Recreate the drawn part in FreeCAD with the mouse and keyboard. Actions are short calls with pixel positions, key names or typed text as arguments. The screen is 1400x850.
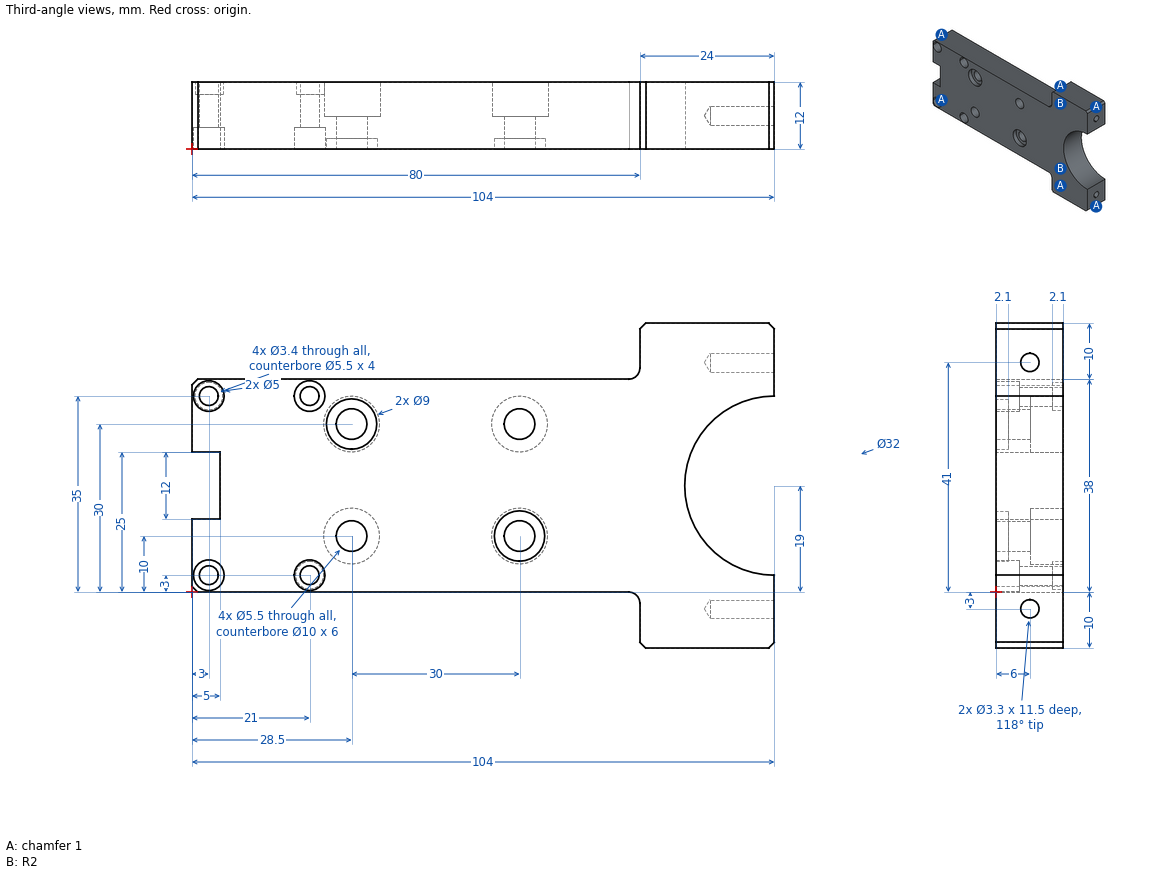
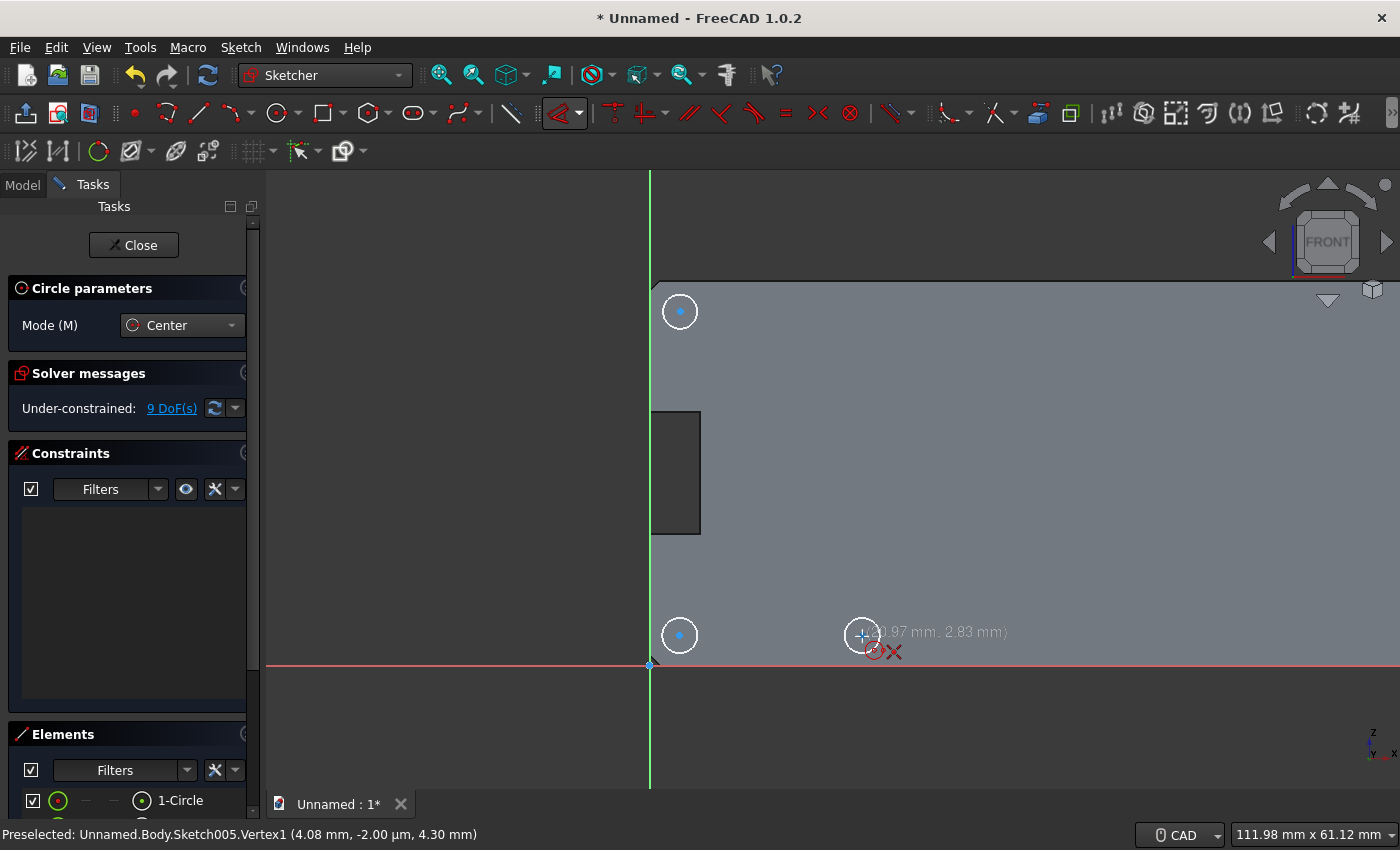
scroll(862, 311, up, 2)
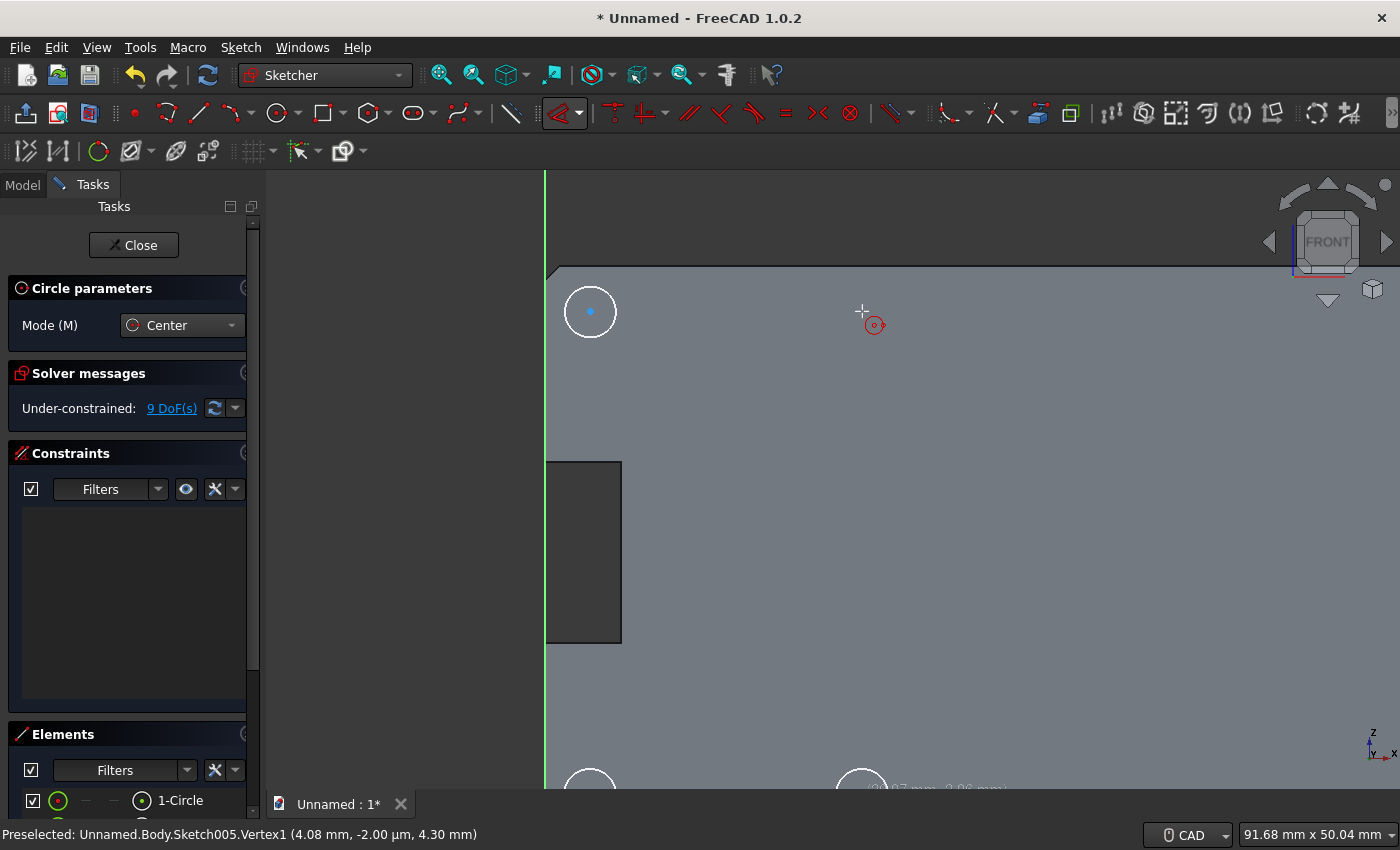
click(862, 311)
click(881, 293)
key(Escape)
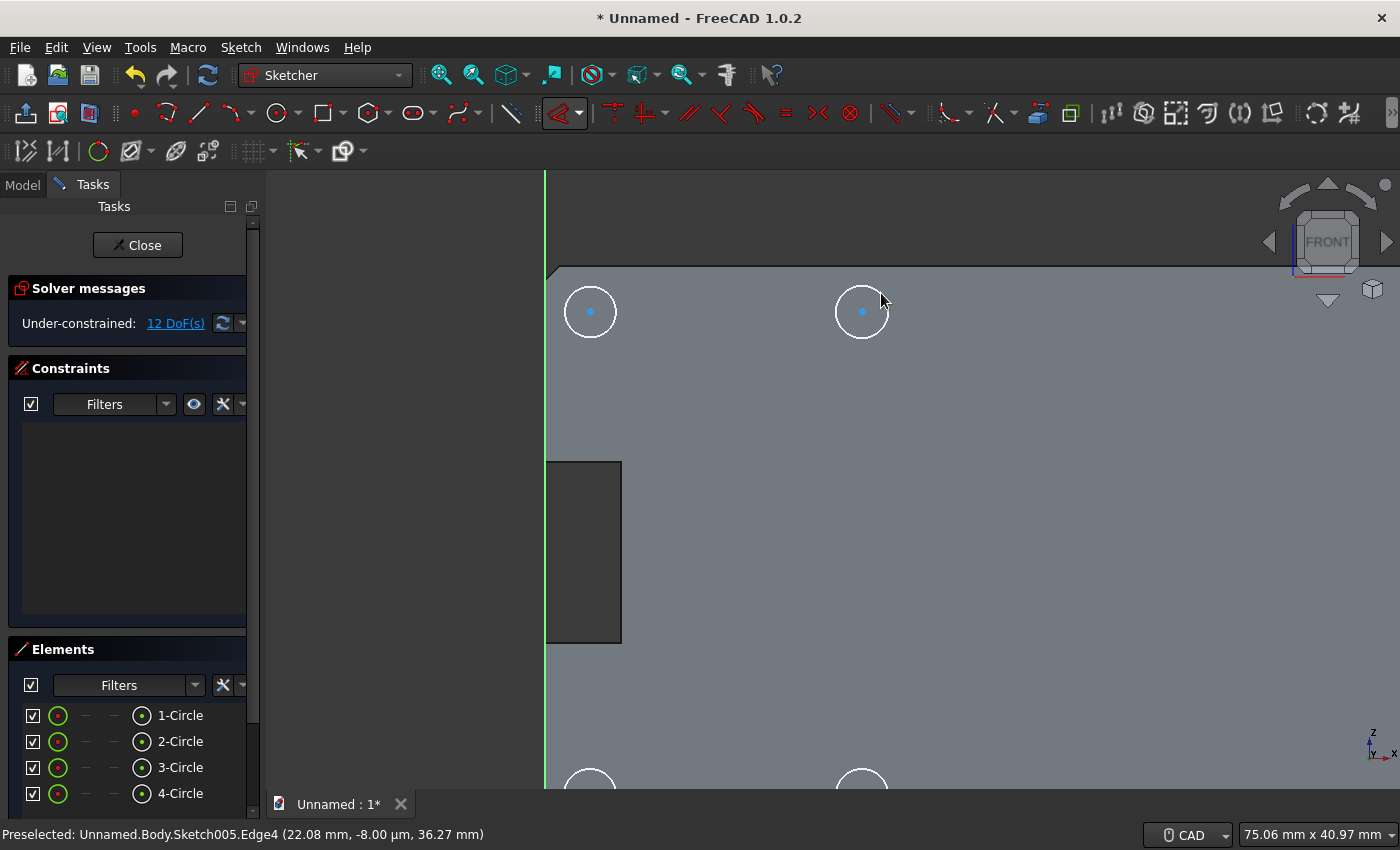
click(608, 294)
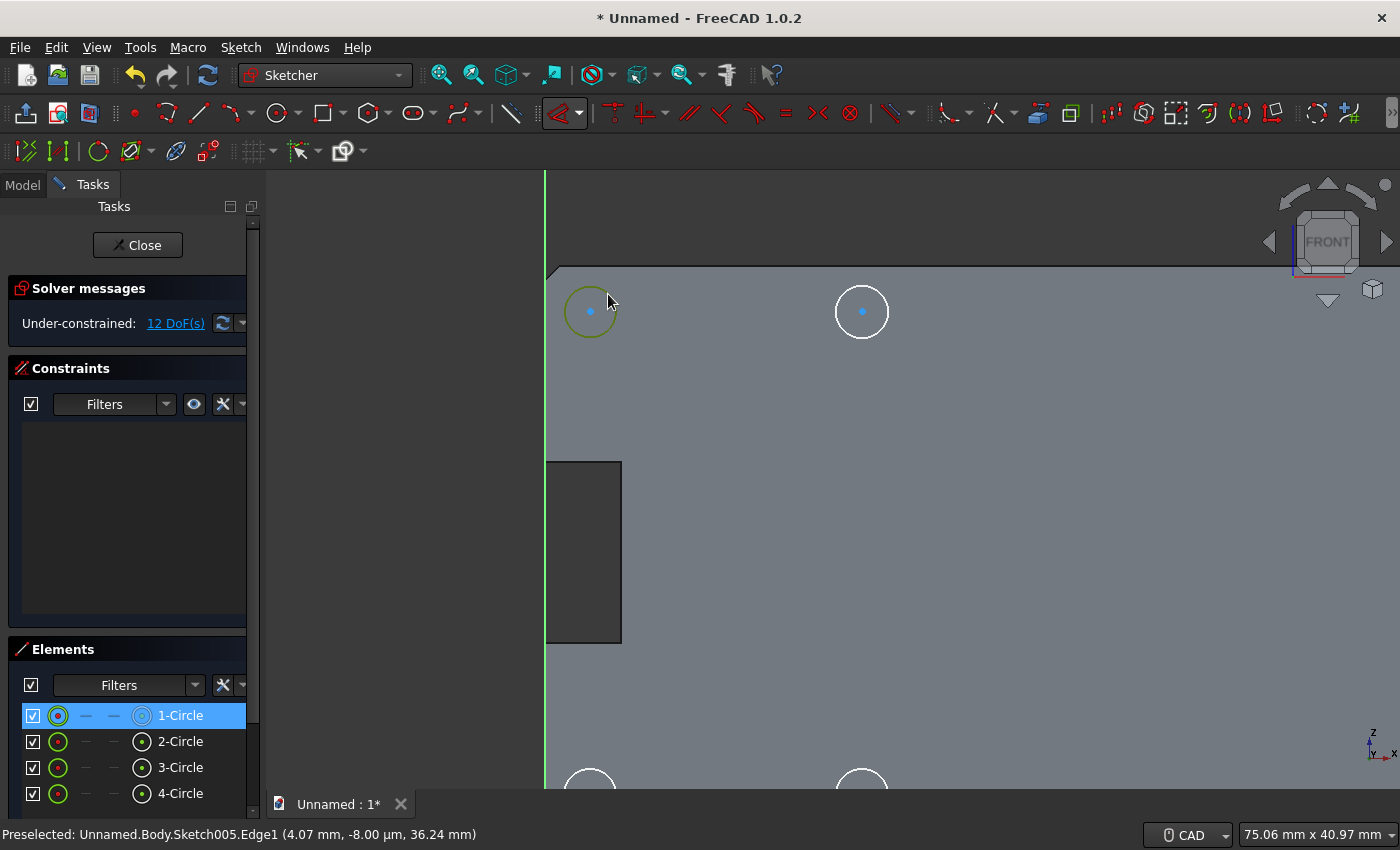
scroll(862, 310, down, 2)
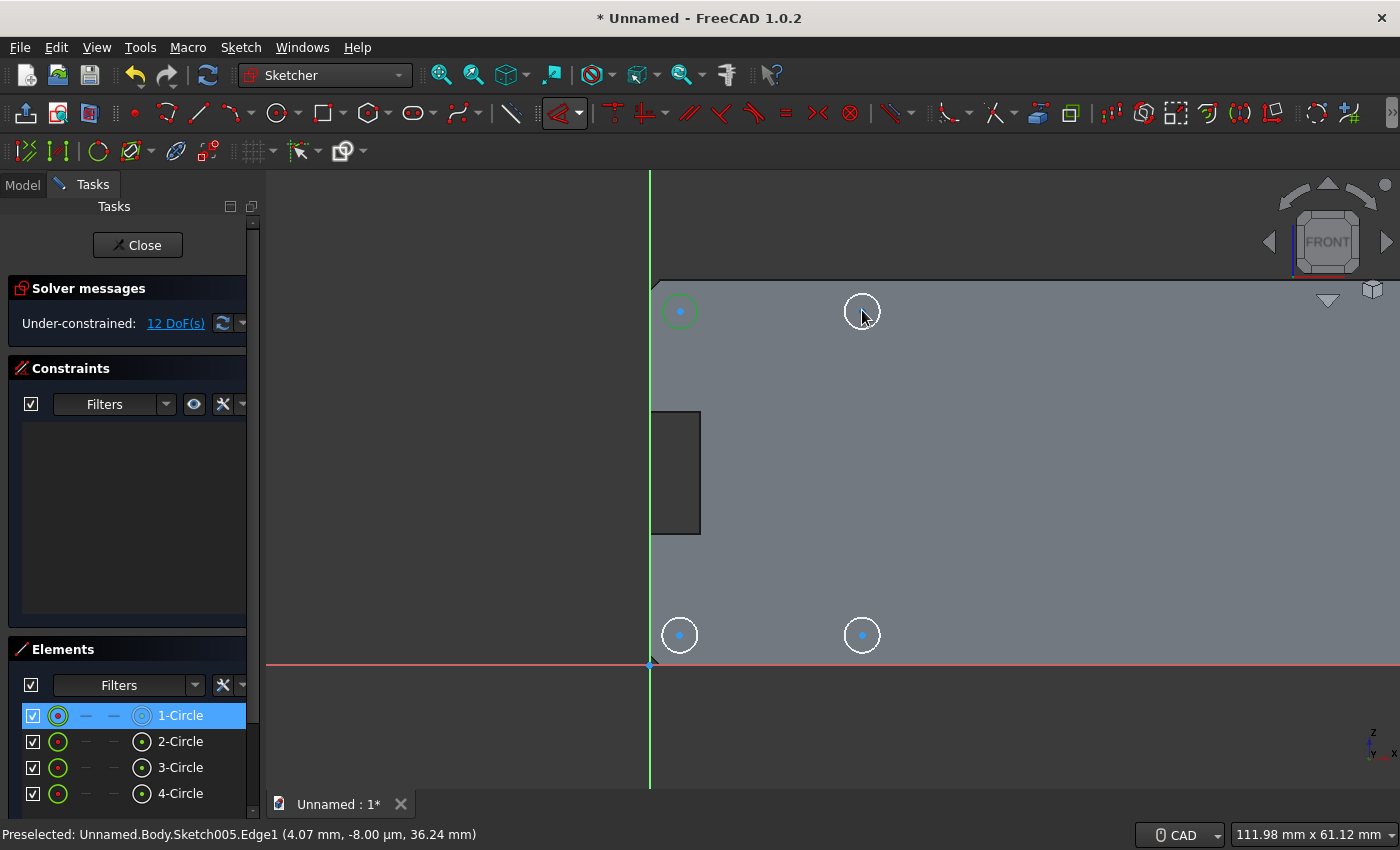
click(875, 623)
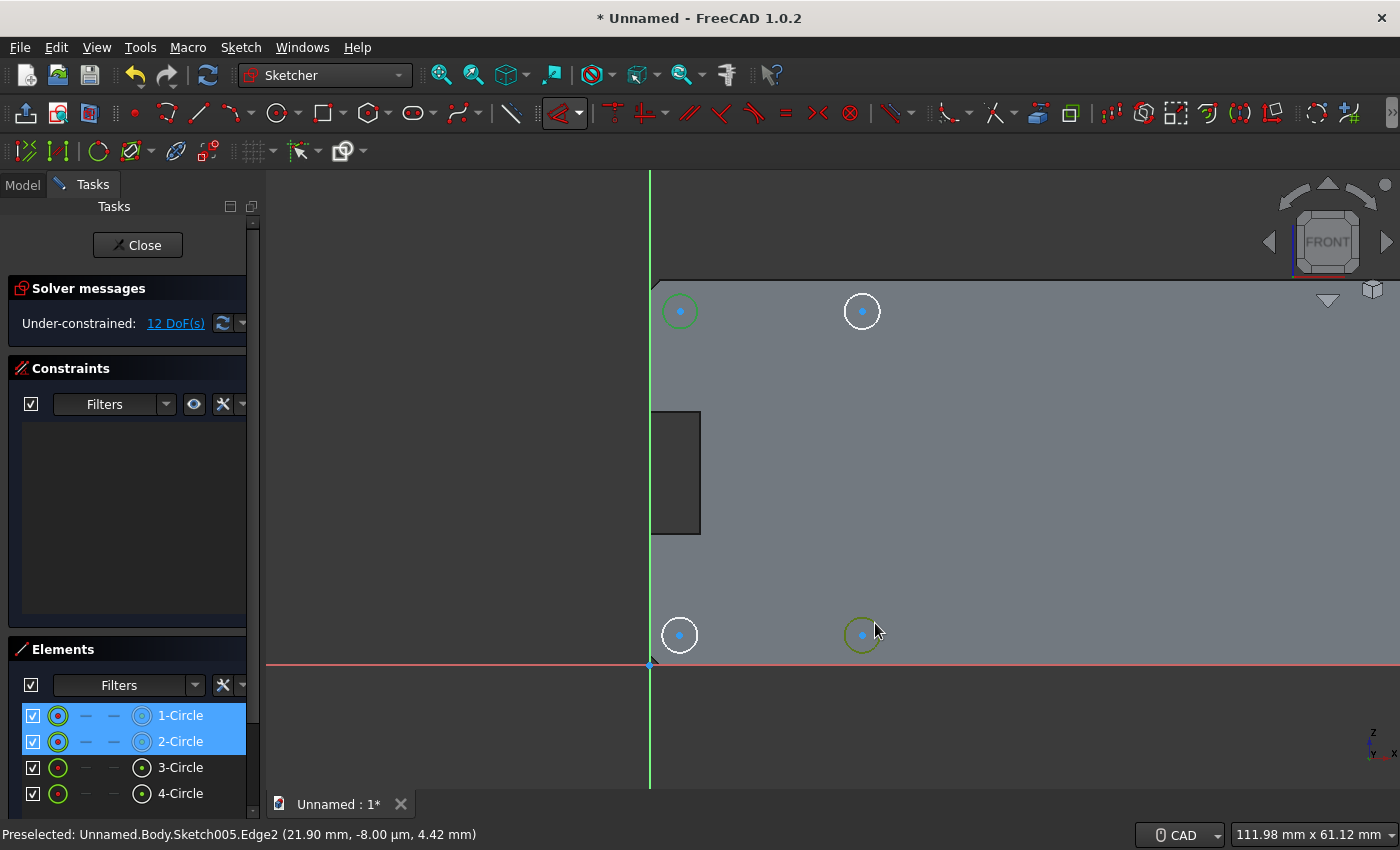
click(692, 623)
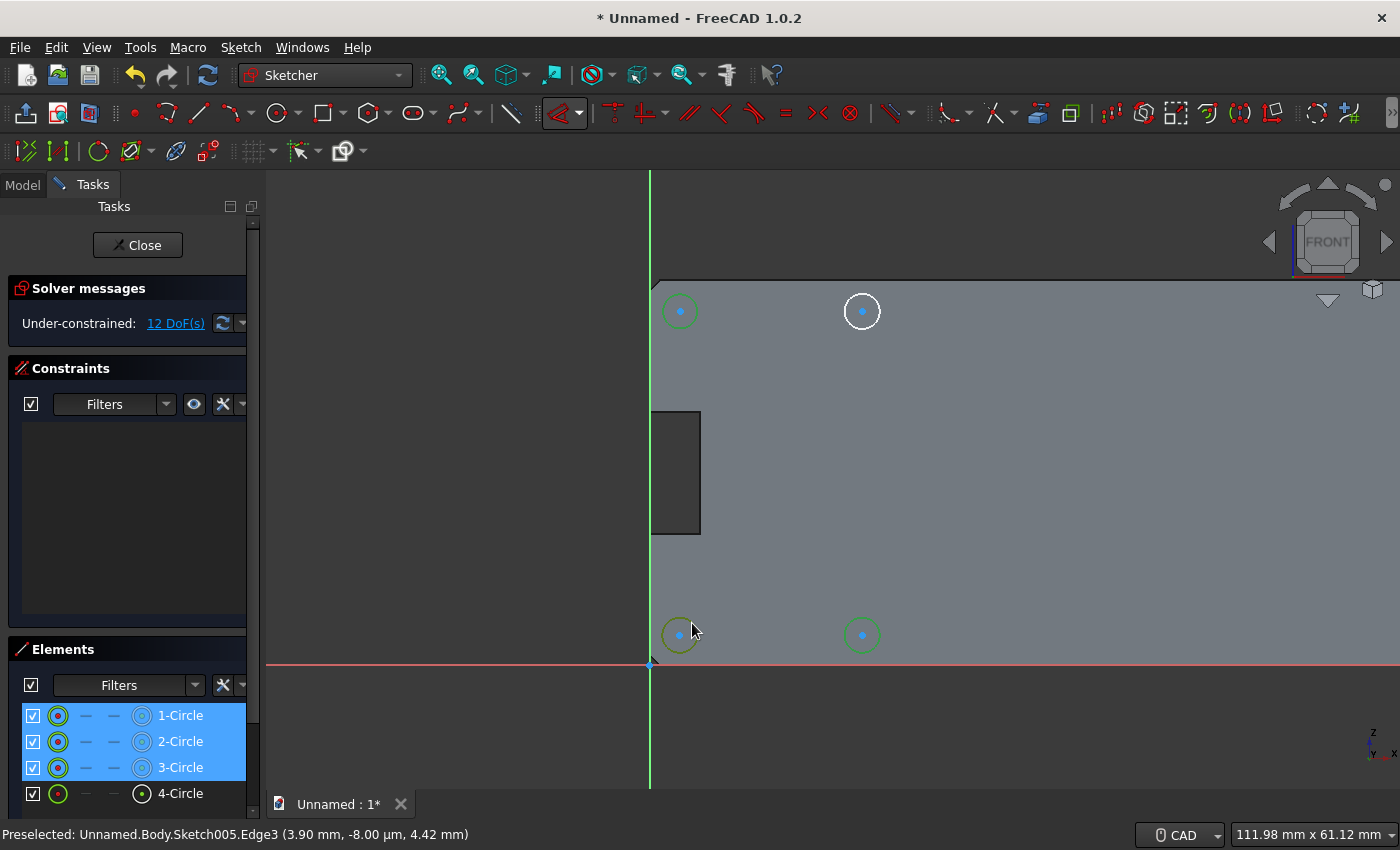
click(875, 299)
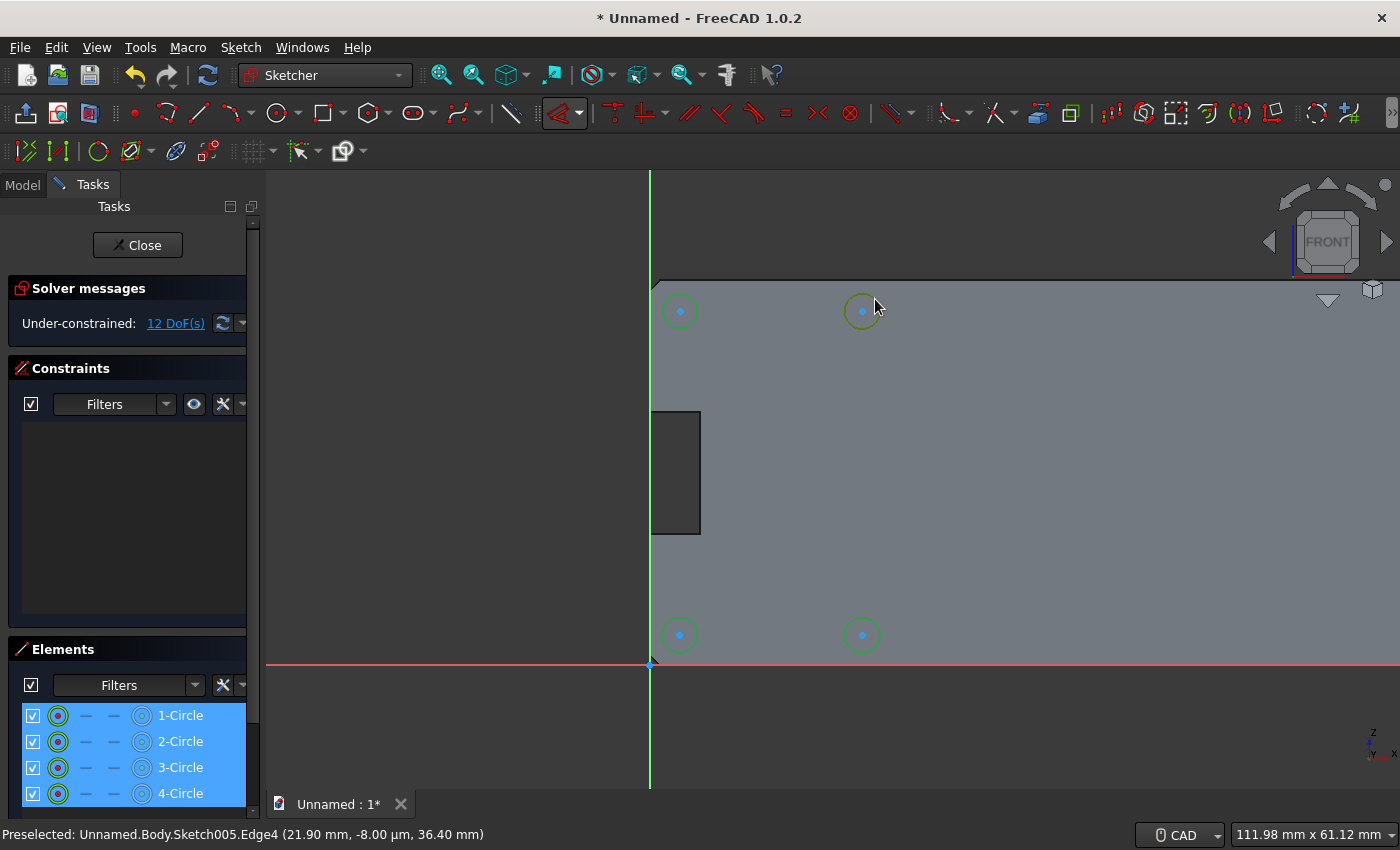
click(786, 114)